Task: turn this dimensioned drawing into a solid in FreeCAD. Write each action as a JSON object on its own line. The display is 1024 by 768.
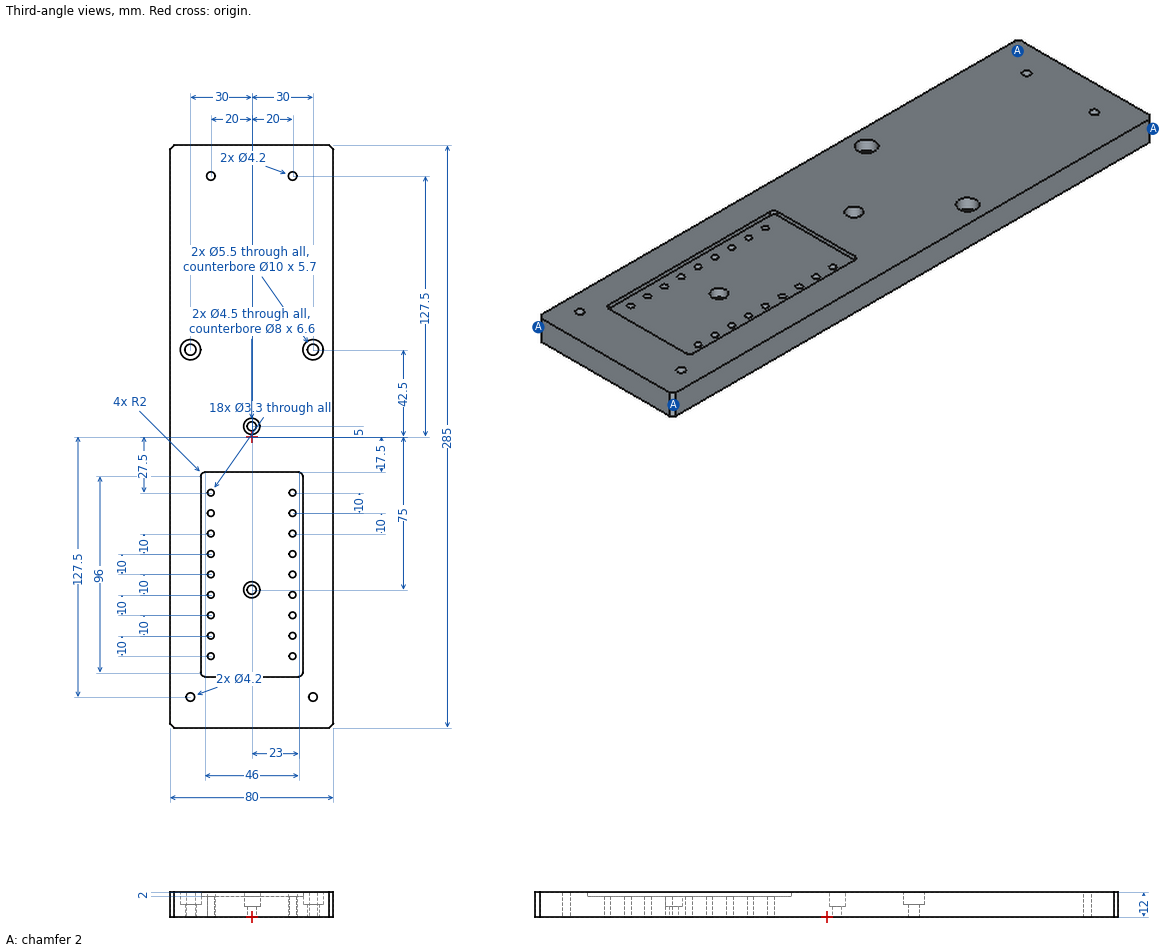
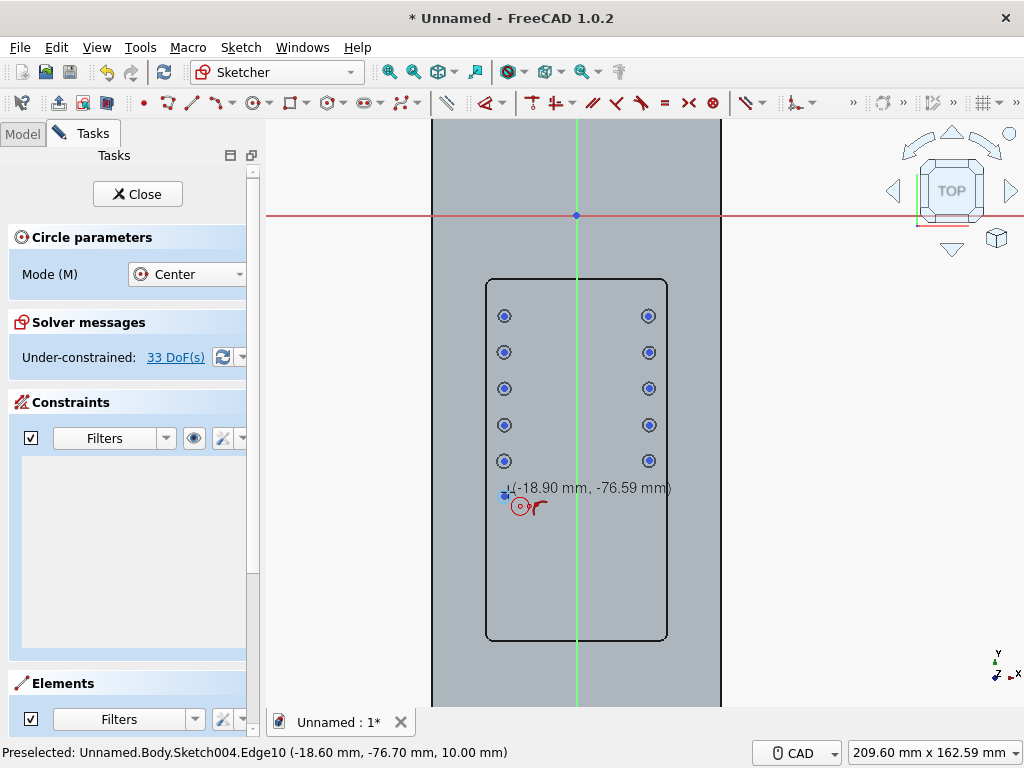
{"action": "scroll", "coordinate": [649, 496], "scroll_direction": "up", "scroll_amount": 7}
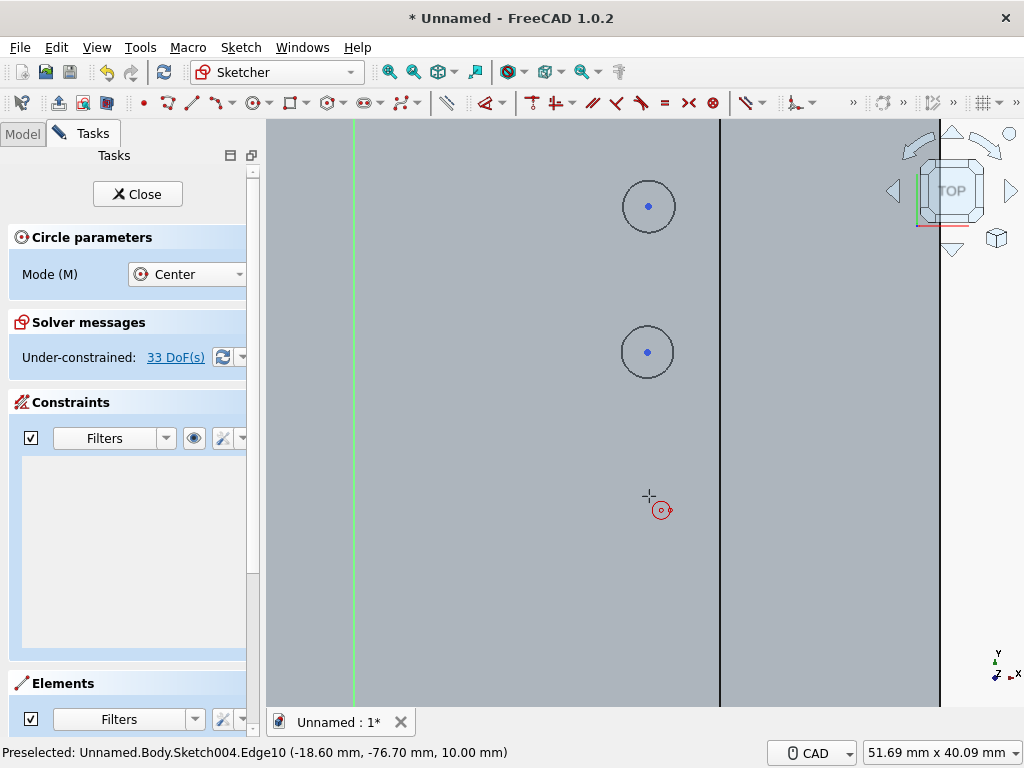
{"action": "scroll", "coordinate": [649, 496], "scroll_direction": "down", "scroll_amount": 7}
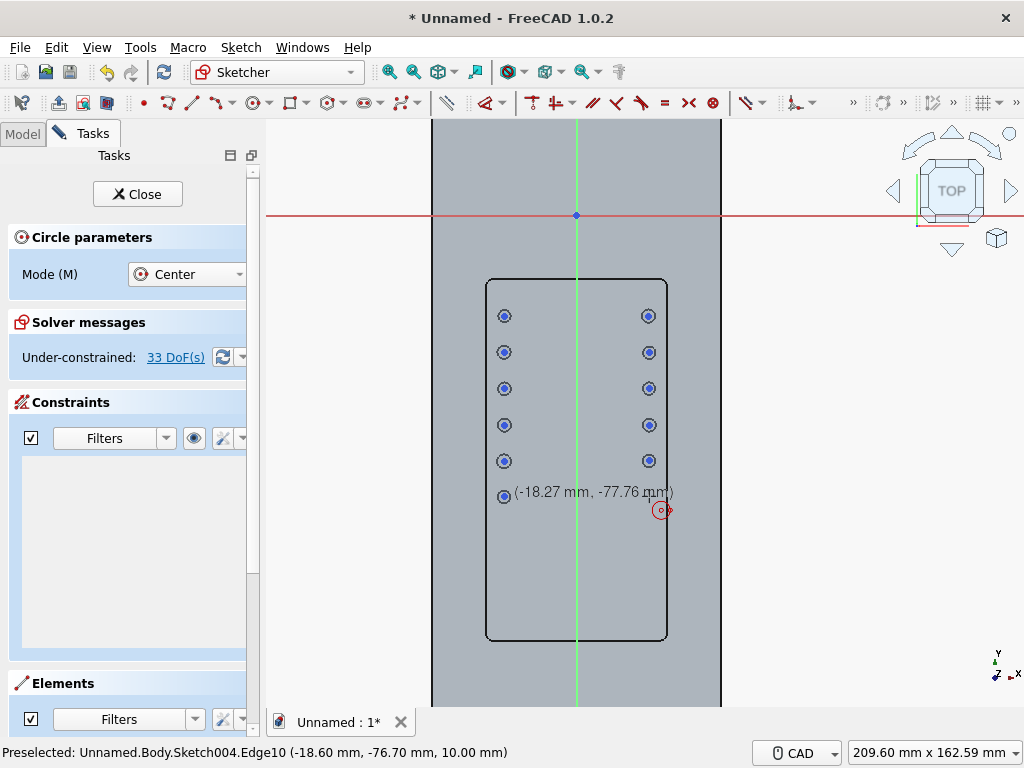
{"action": "left_click", "coordinate": [649, 496]}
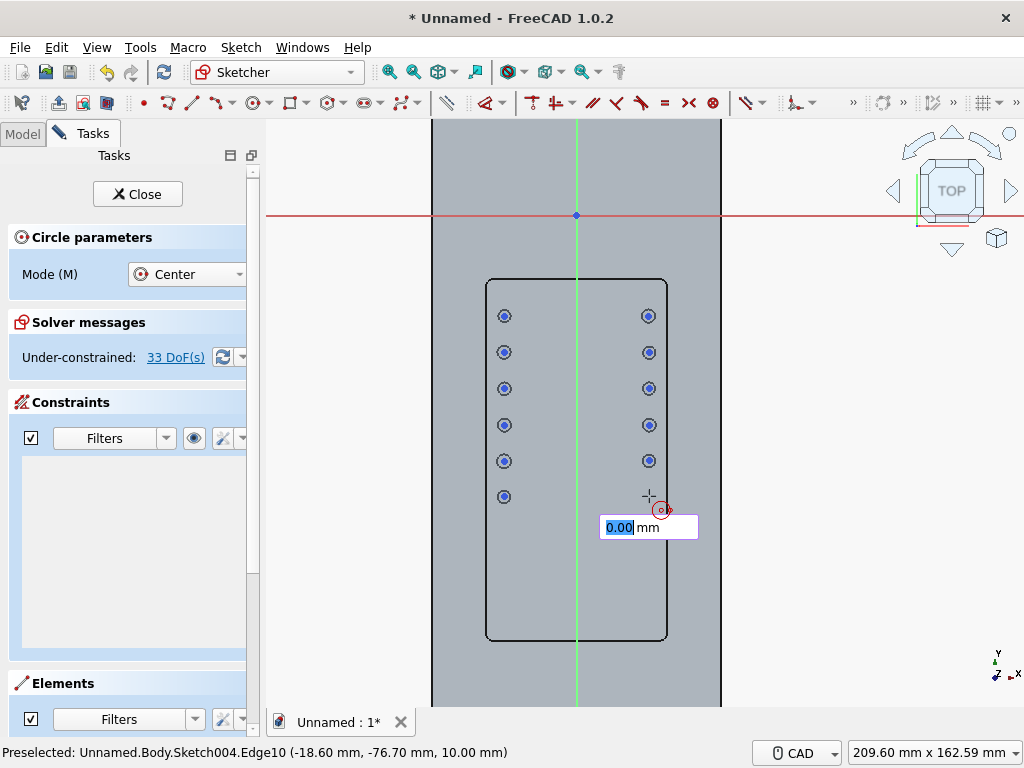
{"action": "scroll", "coordinate": [653, 492], "scroll_direction": "up", "scroll_amount": 5}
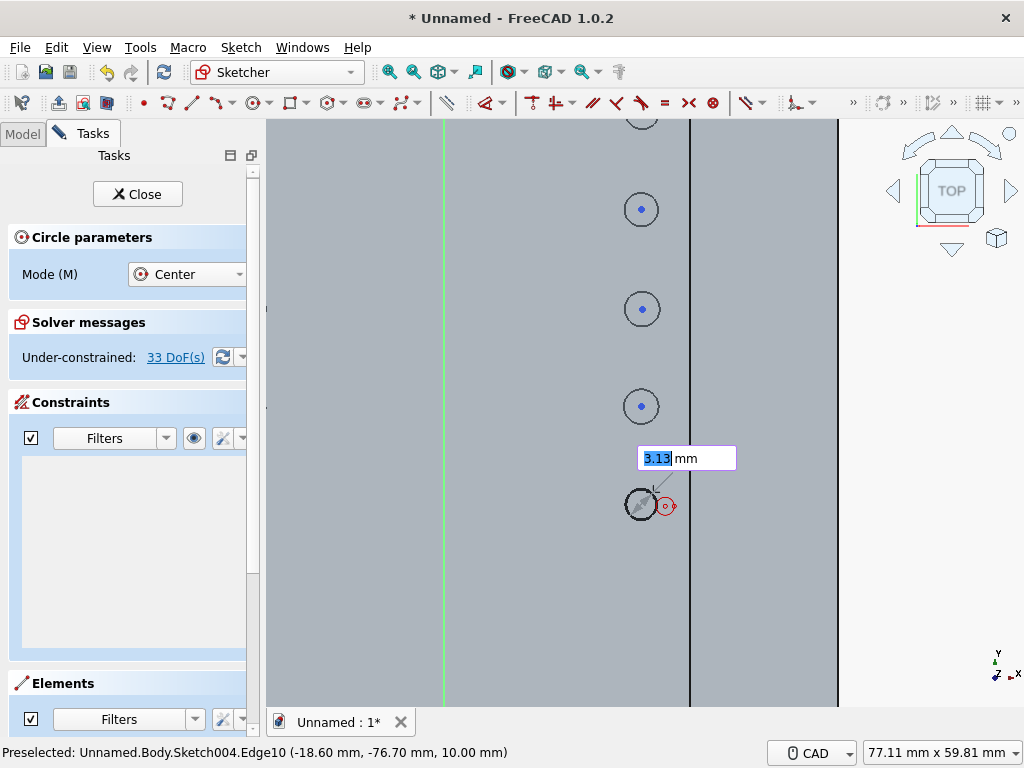
{"action": "left_click", "coordinate": [652, 491]}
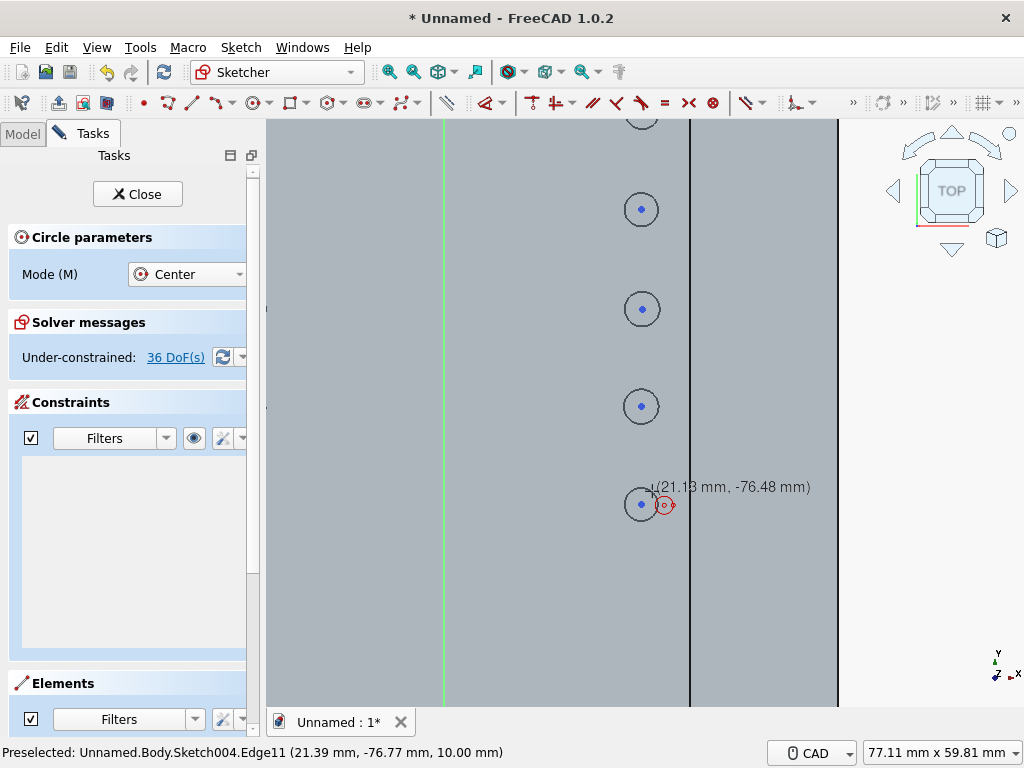
{"action": "scroll", "coordinate": [653, 492], "scroll_direction": "down", "scroll_amount": 5}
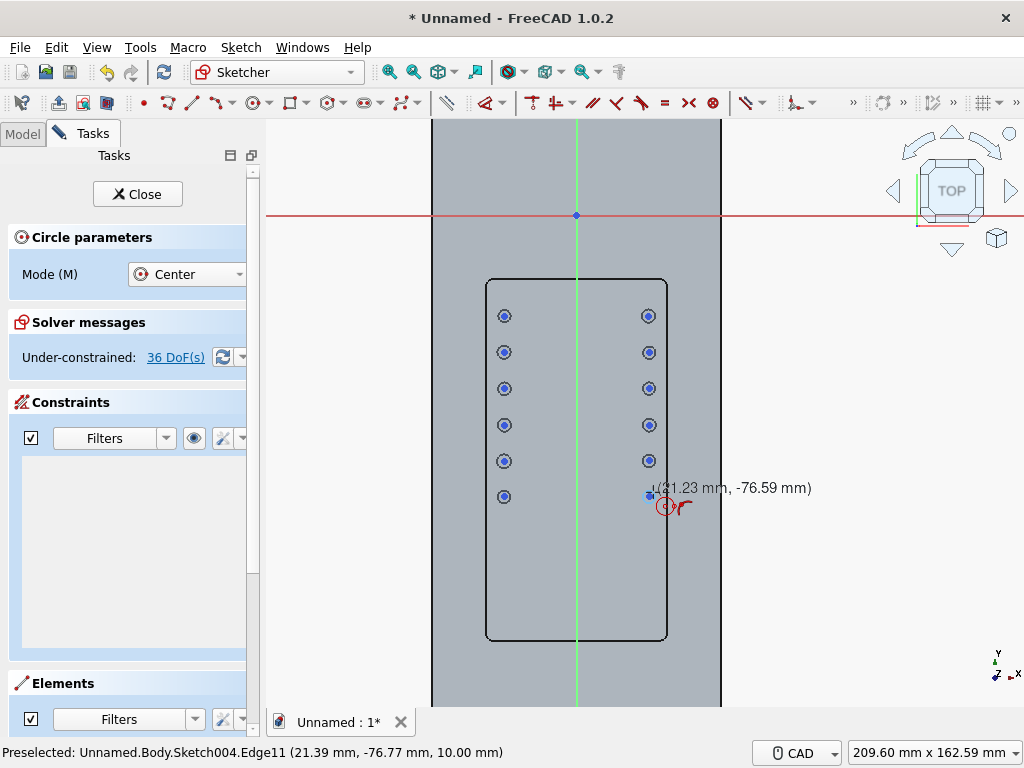
{"action": "scroll", "coordinate": [504, 532], "scroll_direction": "up", "scroll_amount": 7}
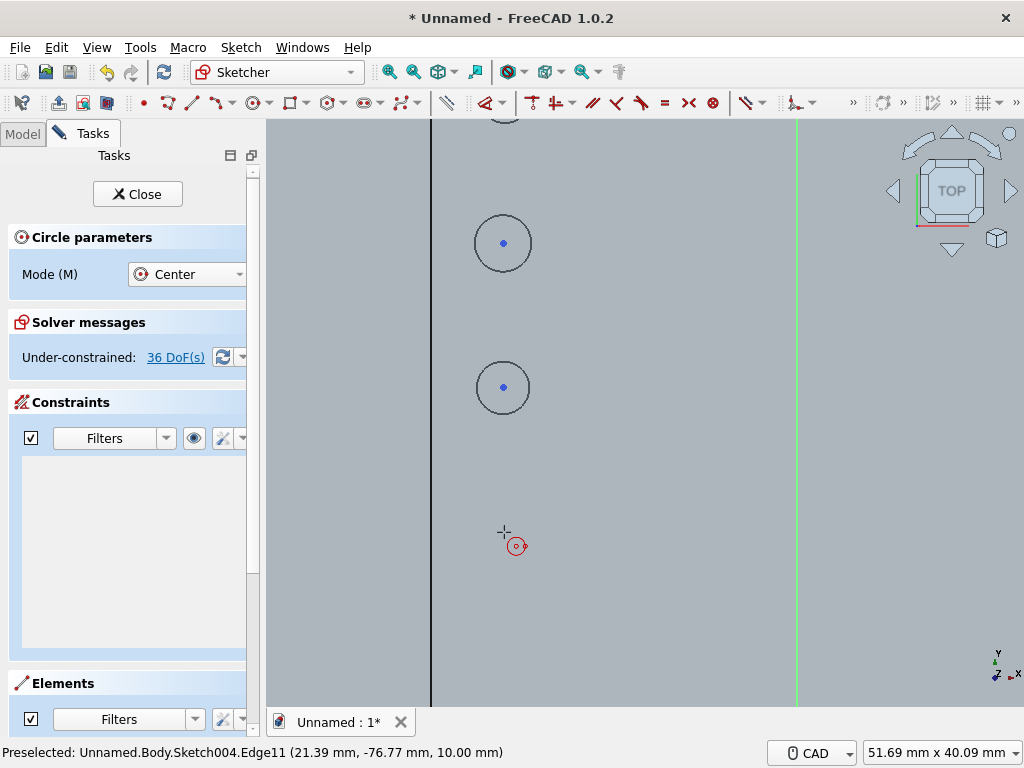
{"action": "scroll", "coordinate": [504, 532], "scroll_direction": "down", "scroll_amount": 7}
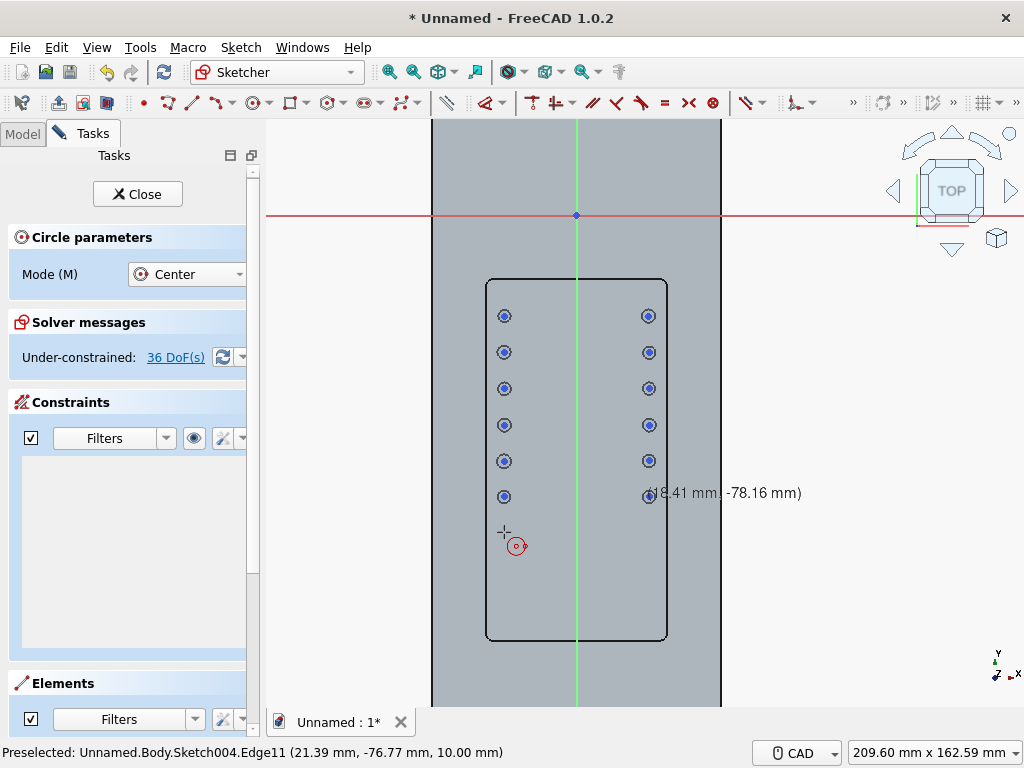
{"action": "left_click", "coordinate": [504, 532]}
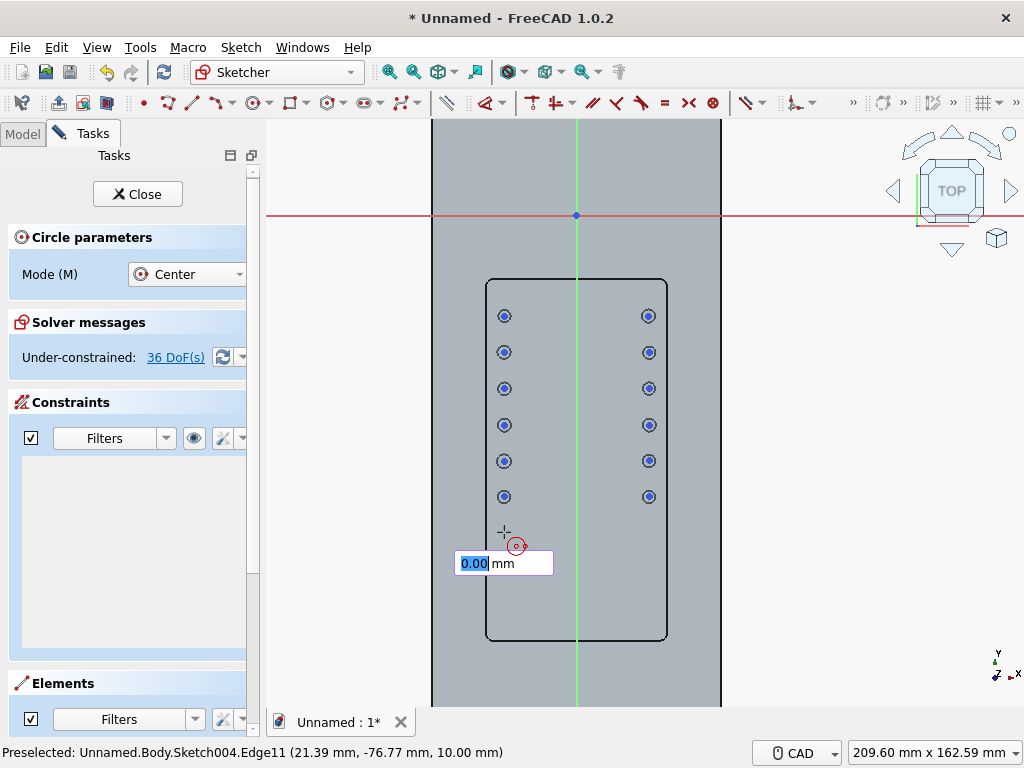
{"action": "scroll", "coordinate": [508, 528], "scroll_direction": "up", "scroll_amount": 5}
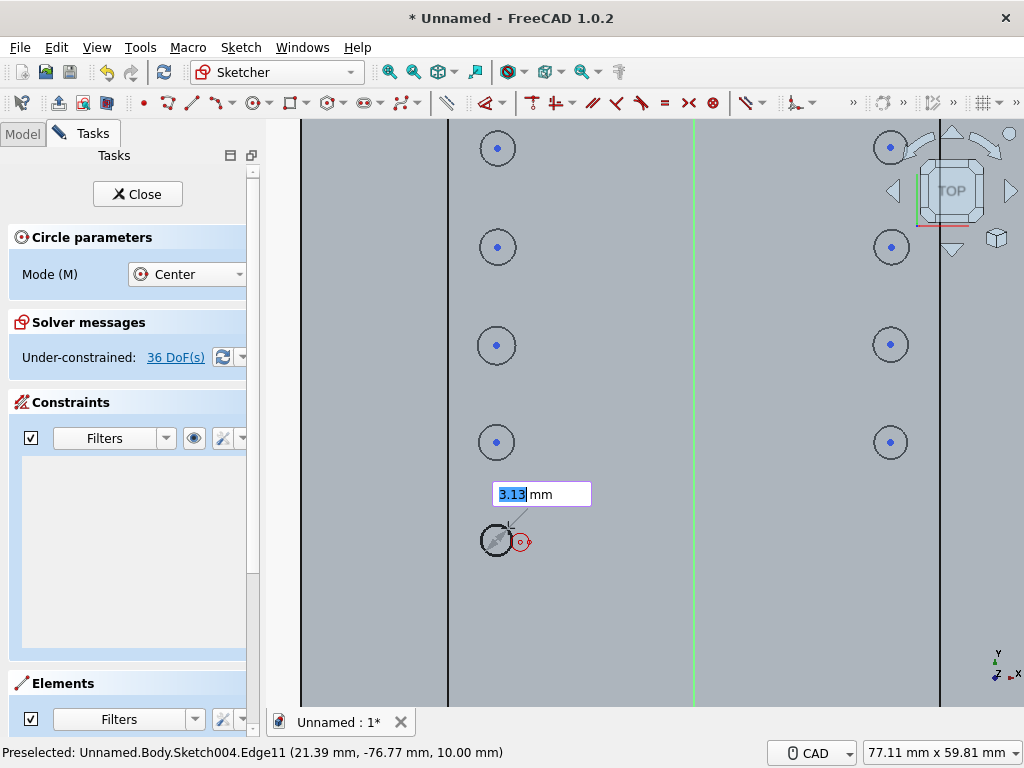
{"action": "left_click", "coordinate": [509, 527]}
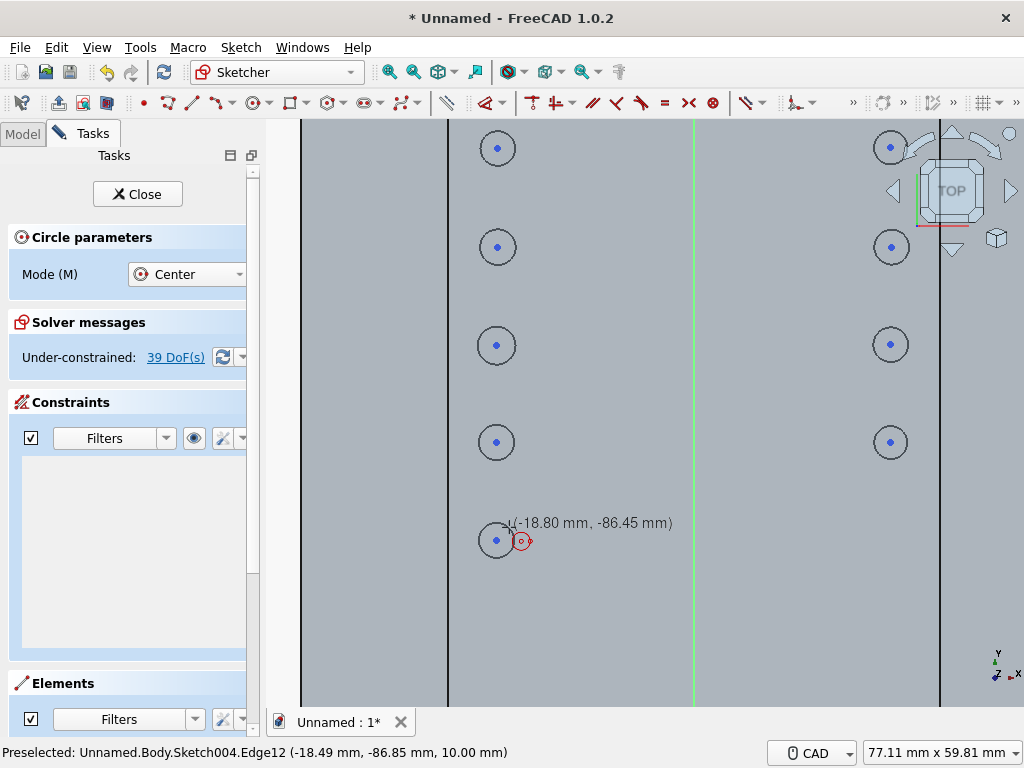
{"action": "scroll", "coordinate": [508, 528], "scroll_direction": "down", "scroll_amount": 5}